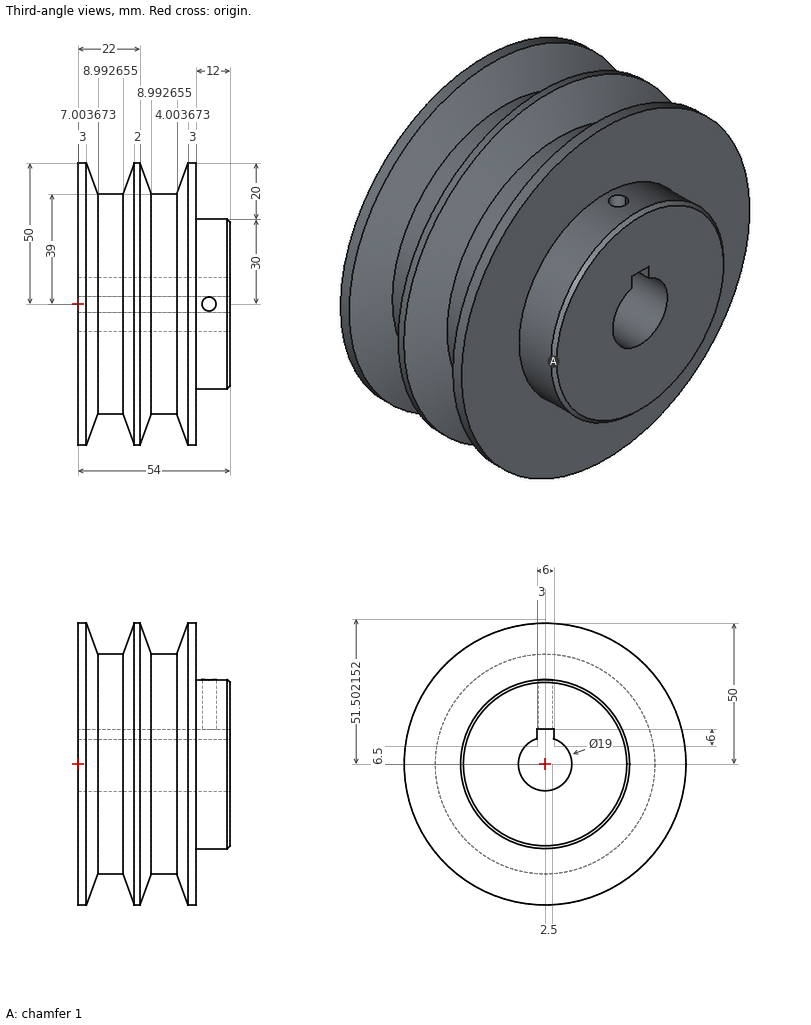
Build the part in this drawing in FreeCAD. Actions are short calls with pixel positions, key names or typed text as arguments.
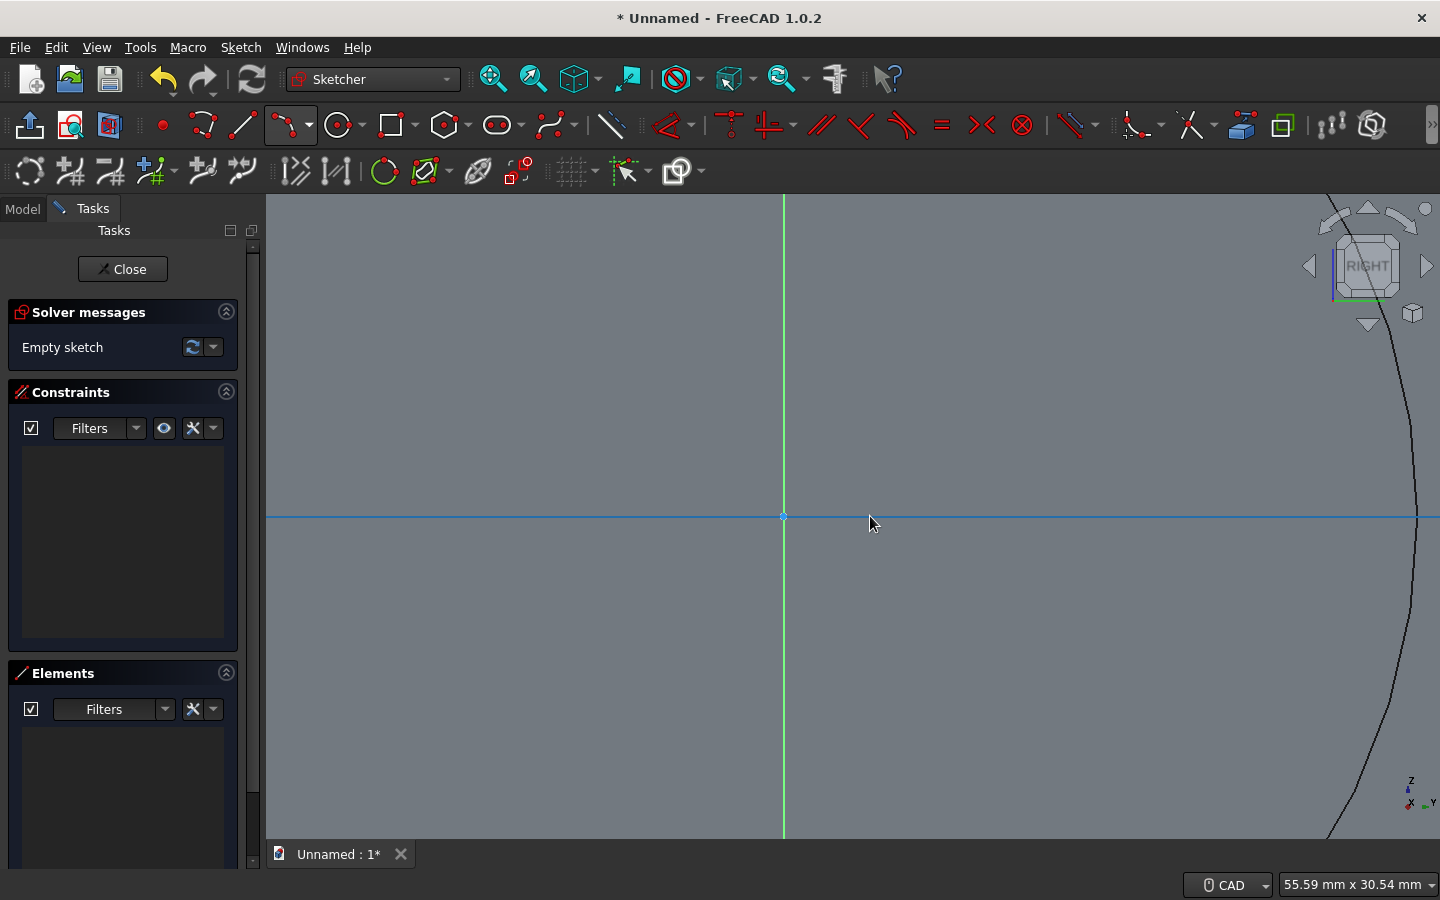
click(338, 126)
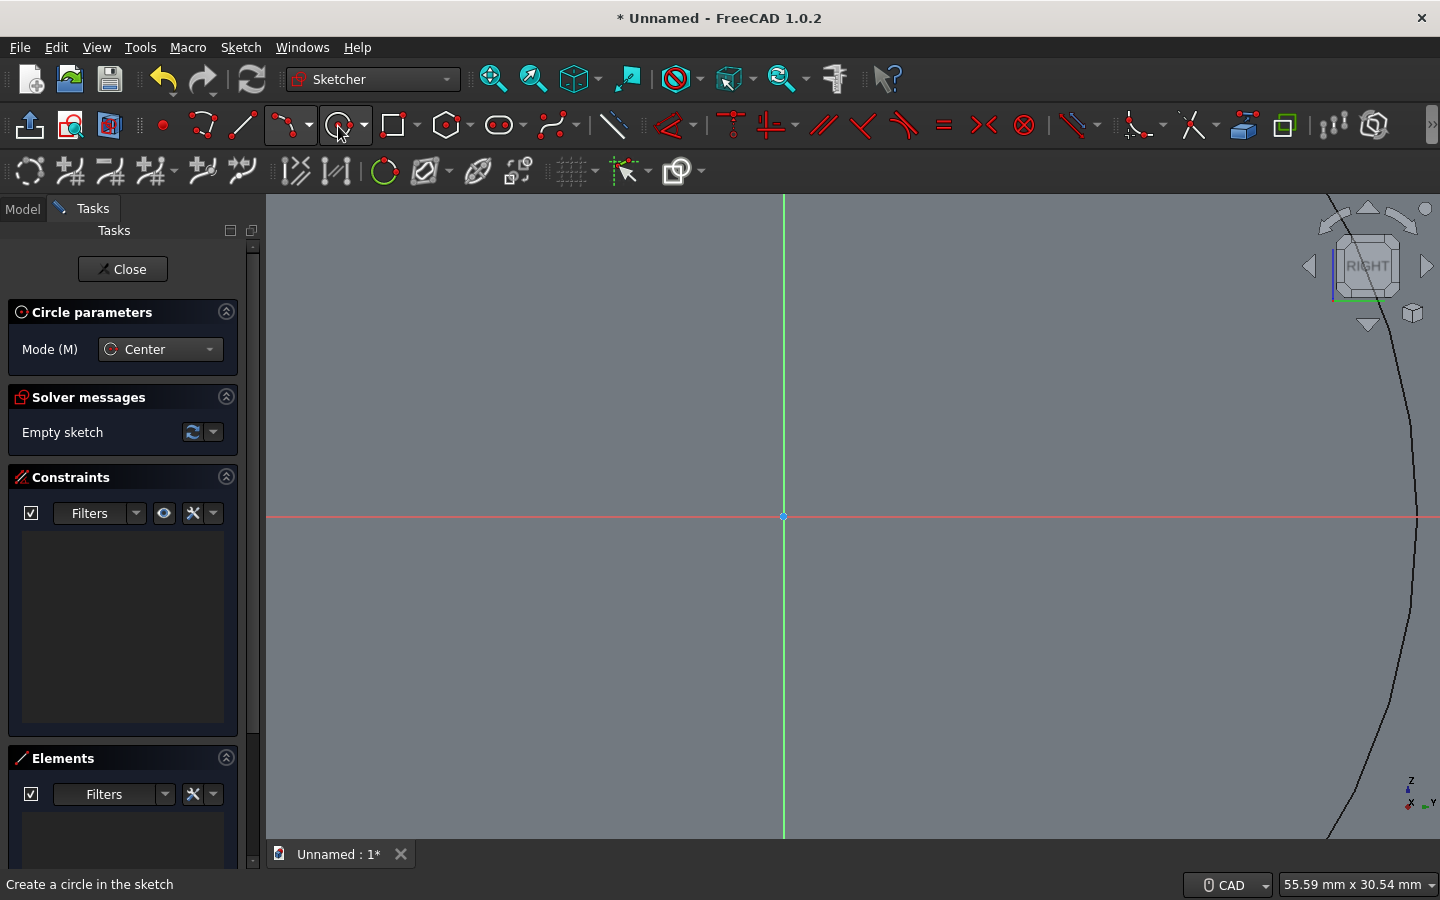
click(784, 516)
move(926, 375)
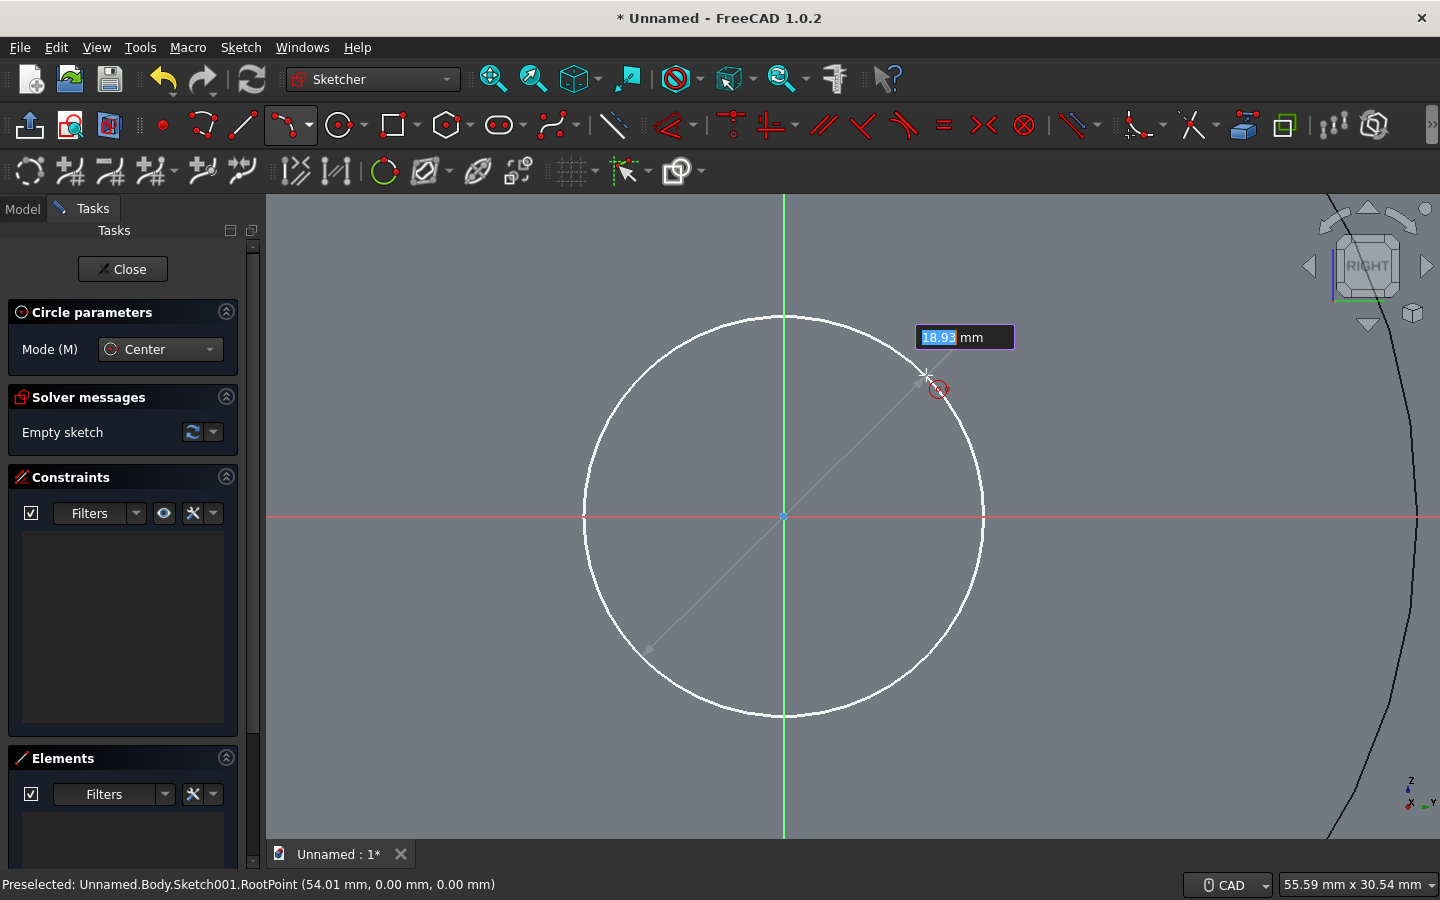
text(19)
key(Return)
key(Escape)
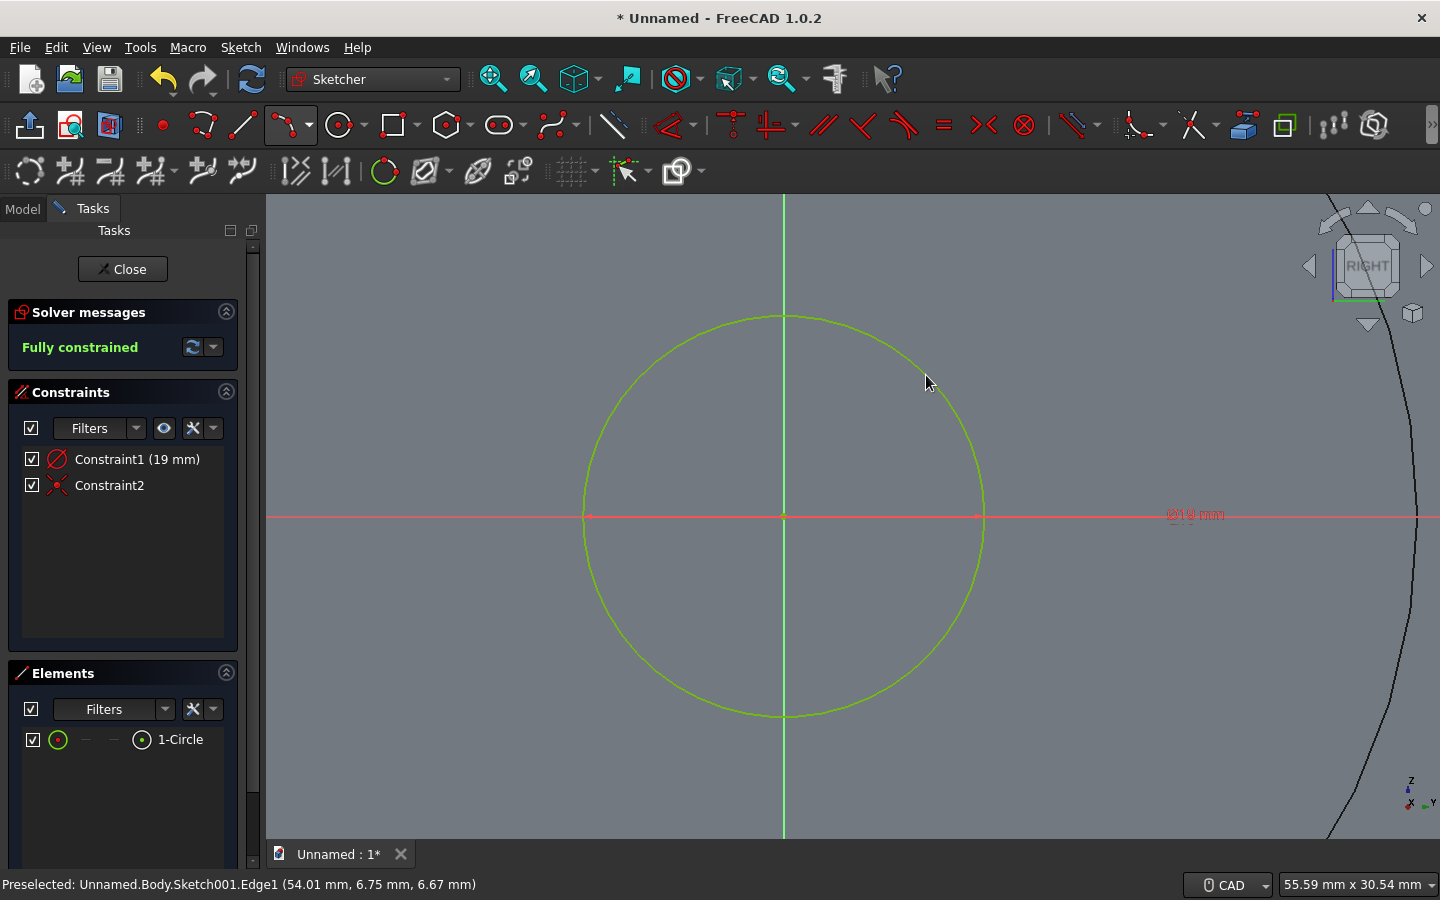
click(123, 269)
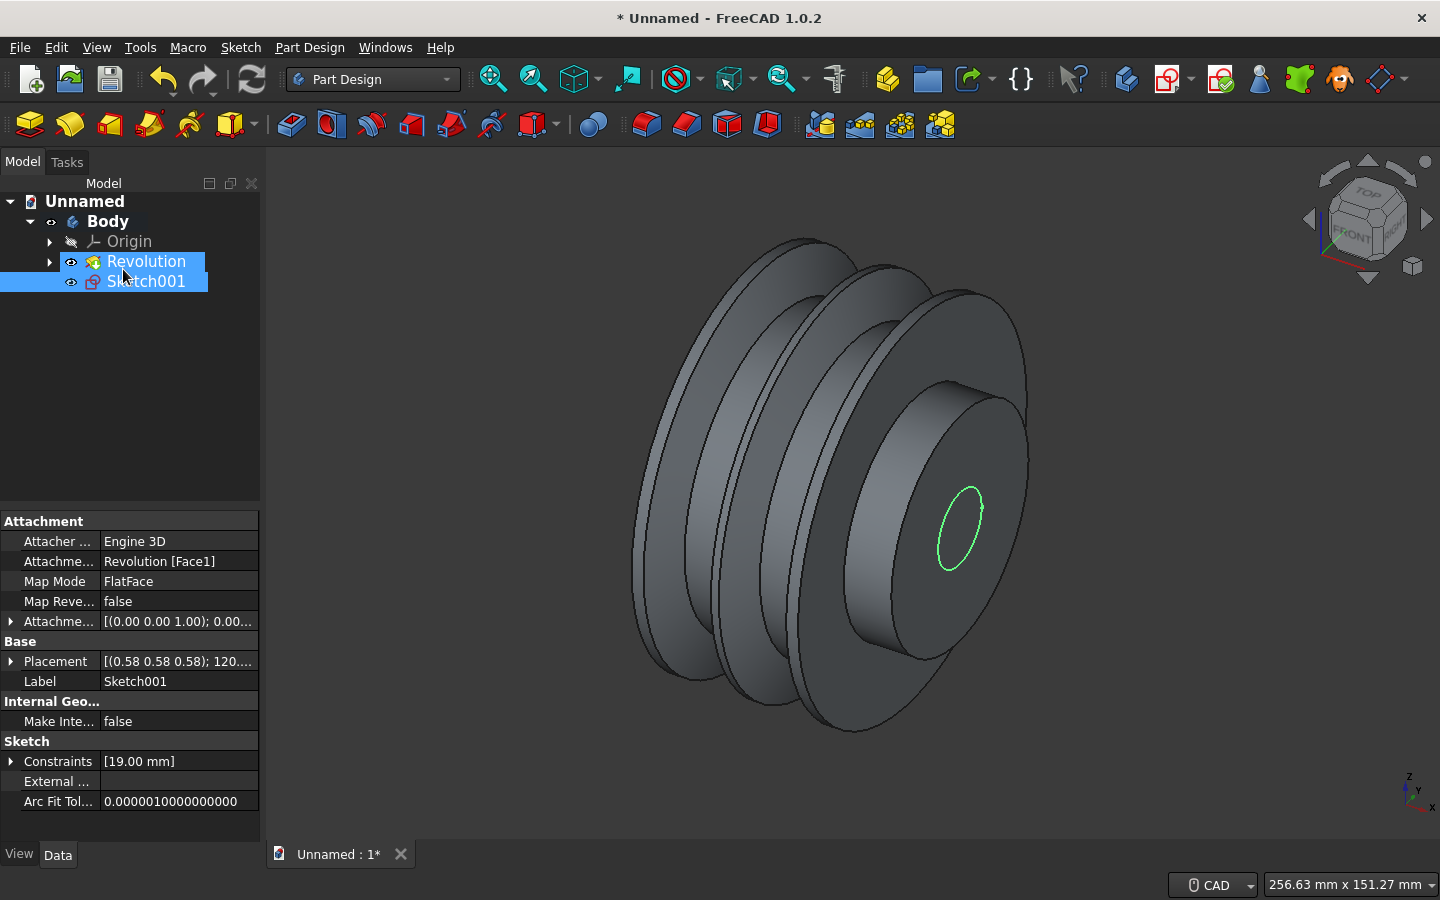
click(292, 124)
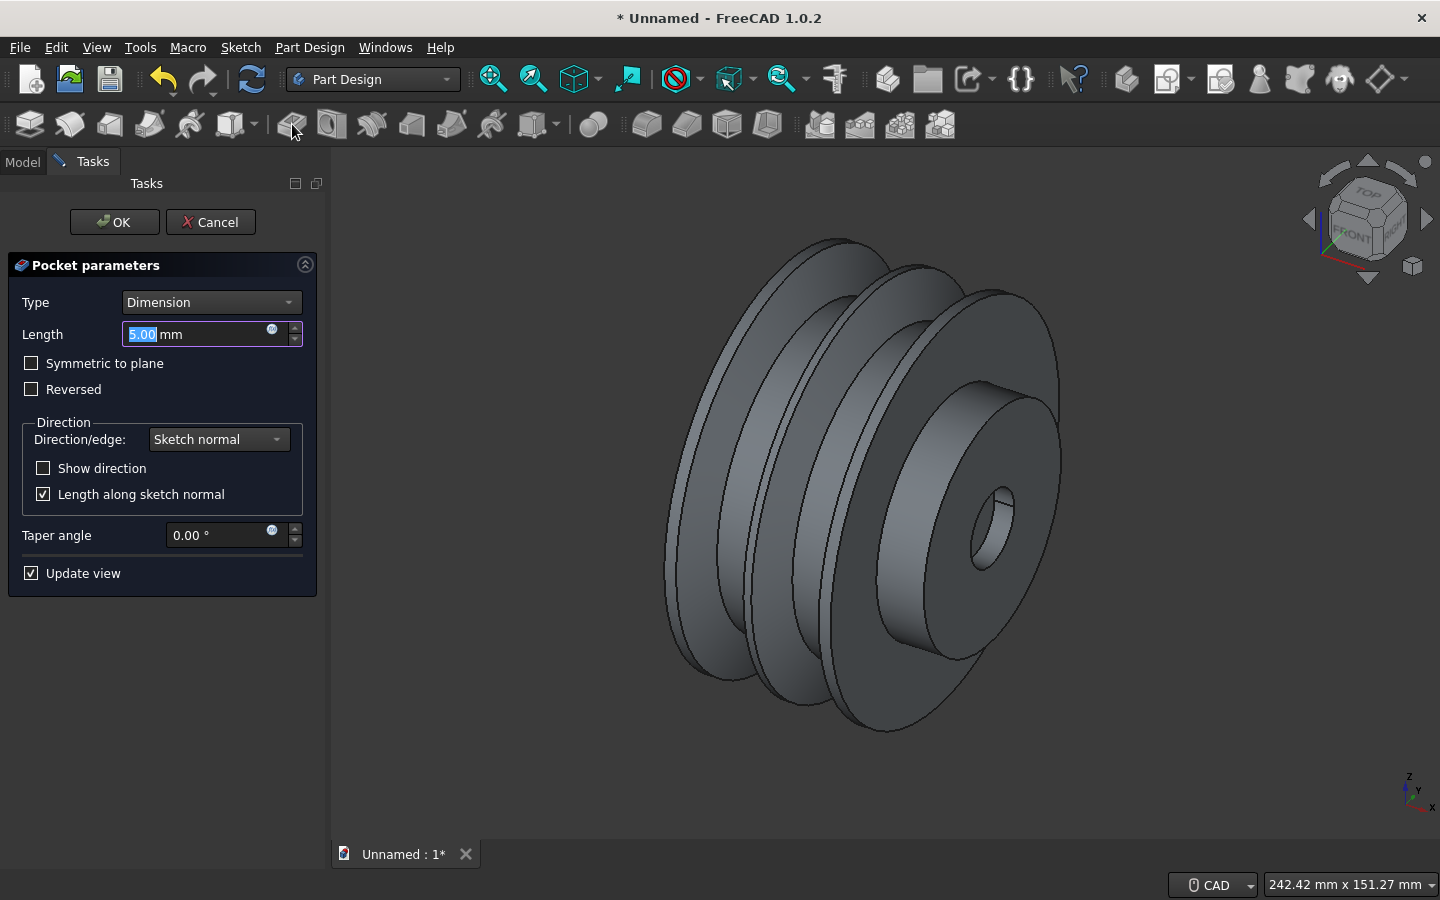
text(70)
key(Tab)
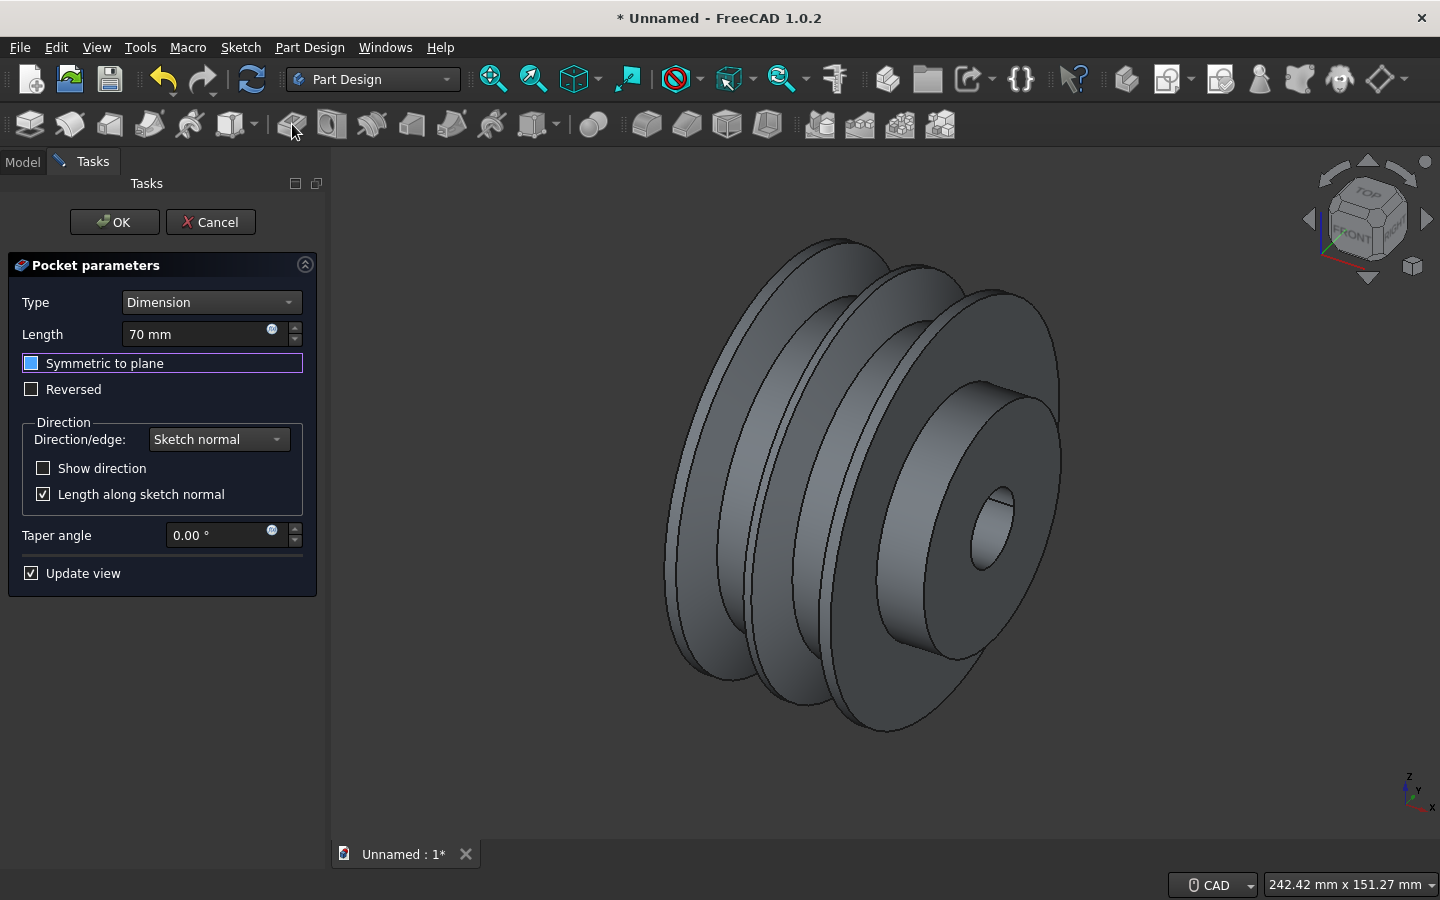
click(115, 222)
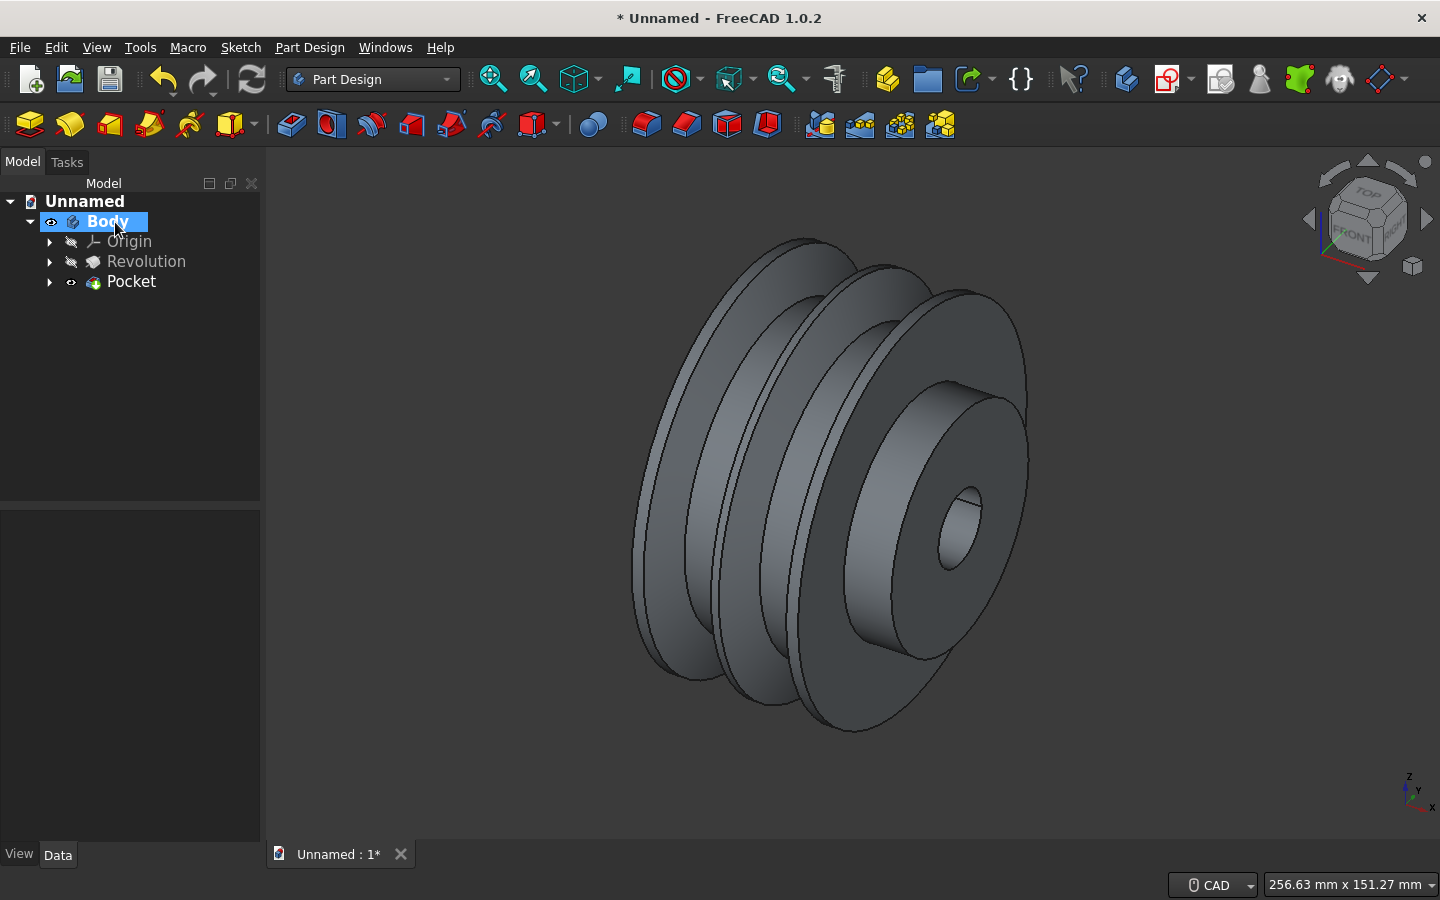
click(50, 242)